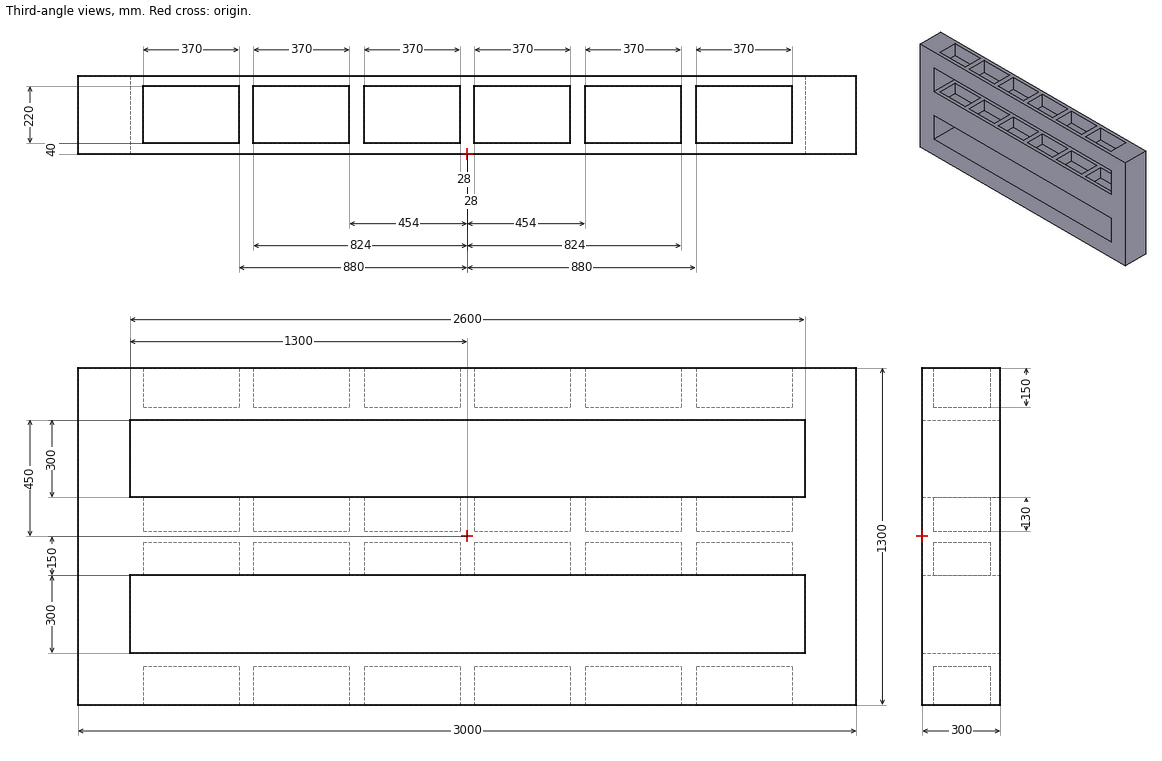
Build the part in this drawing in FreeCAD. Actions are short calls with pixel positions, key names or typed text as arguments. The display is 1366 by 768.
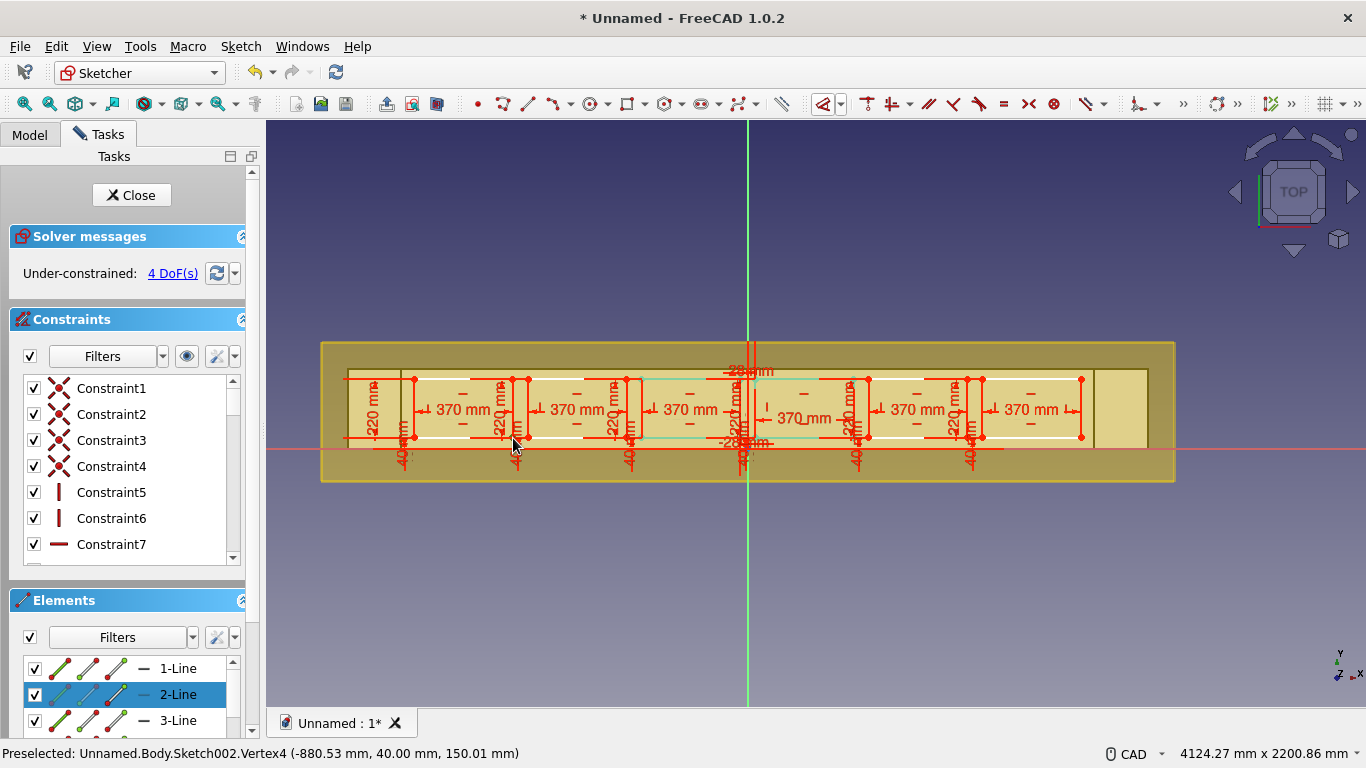
key(l)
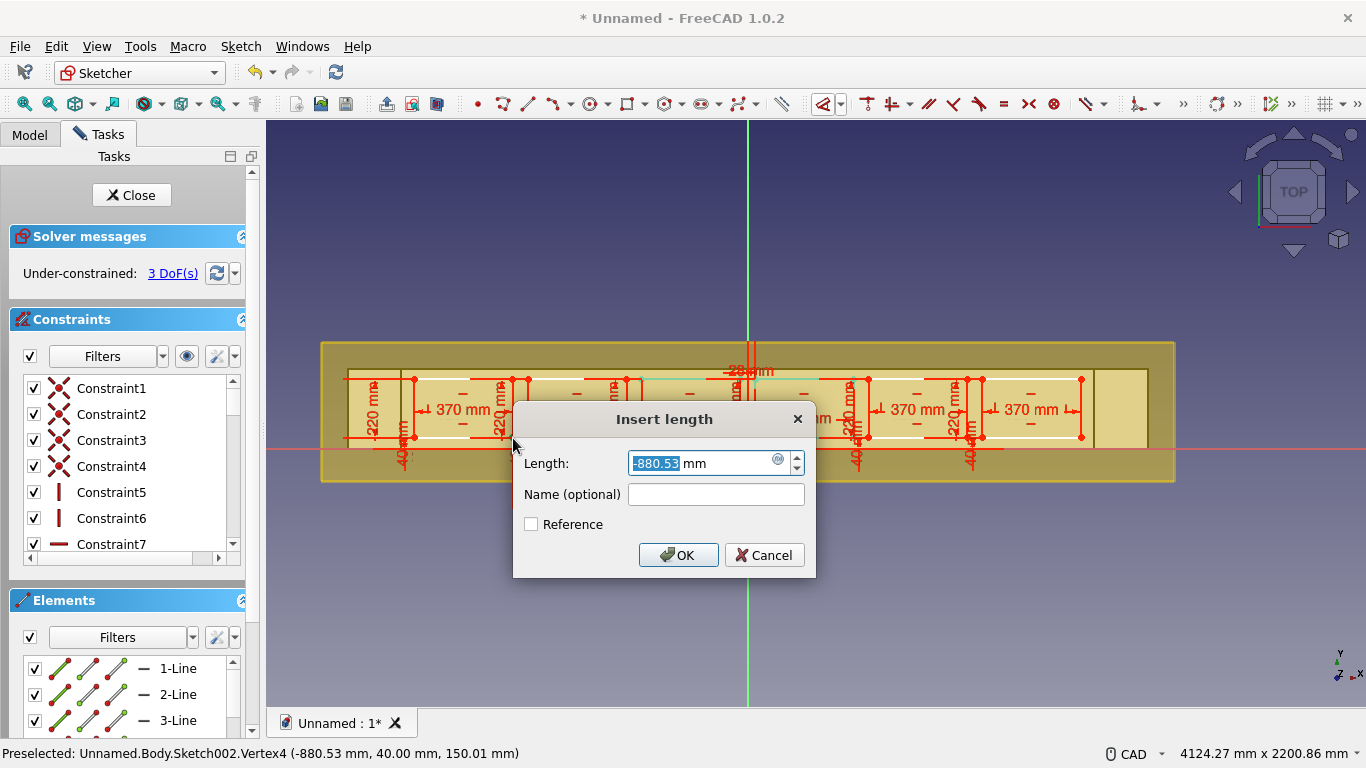
text(-880)
key(Return)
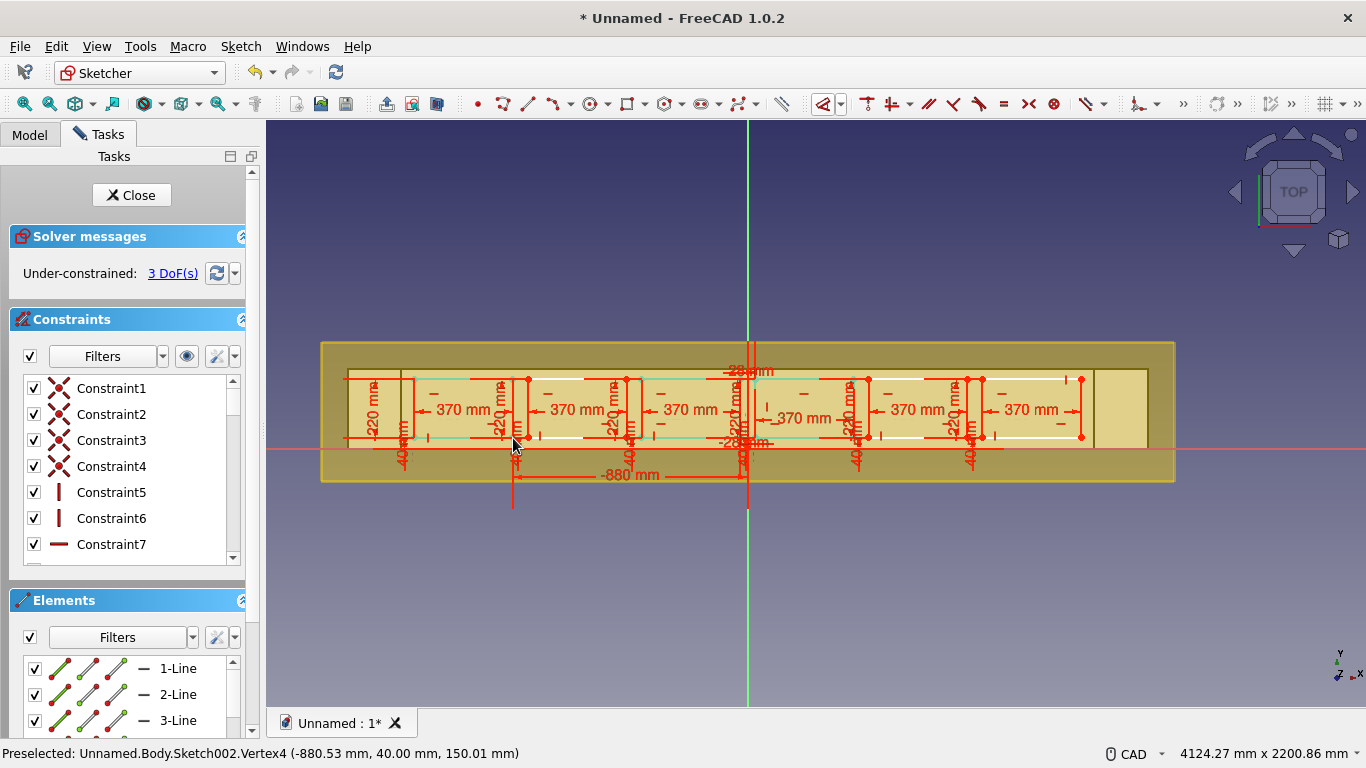
click(528, 379)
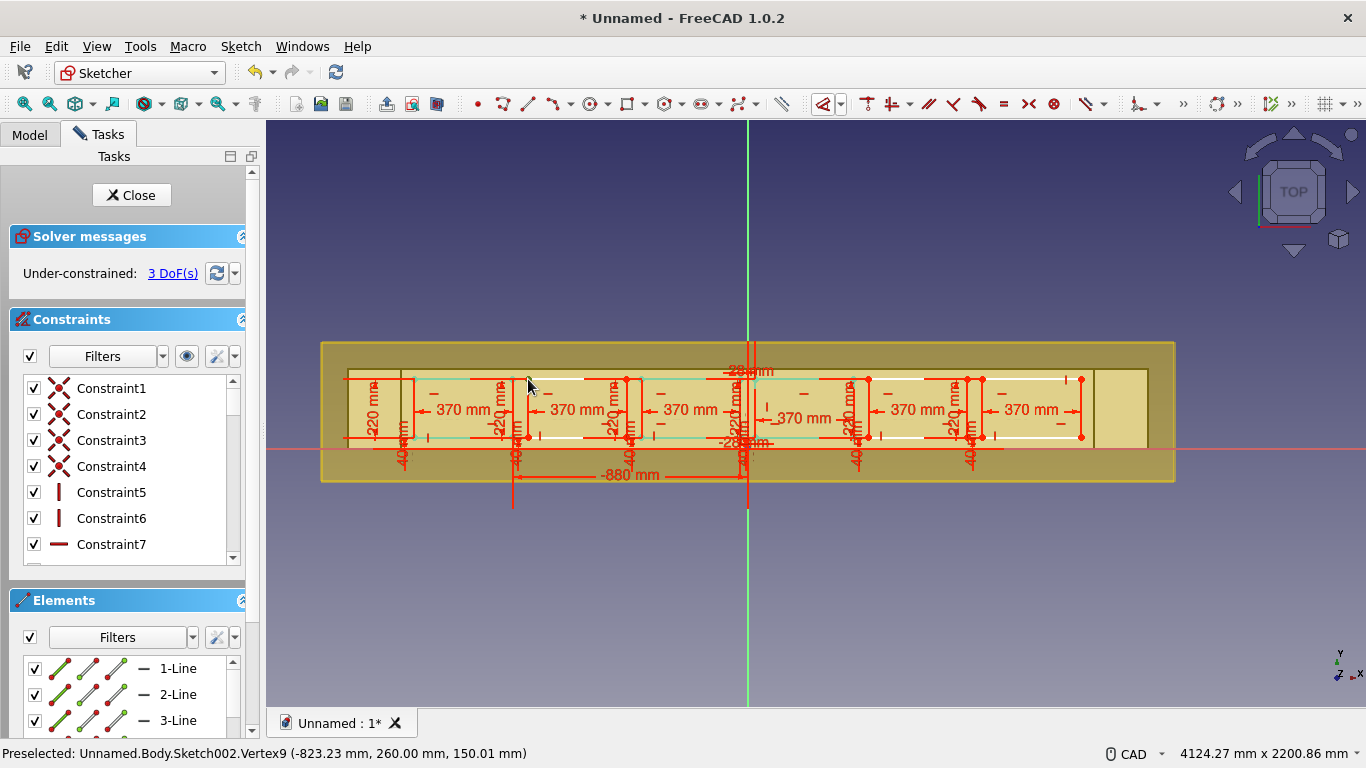
key(l)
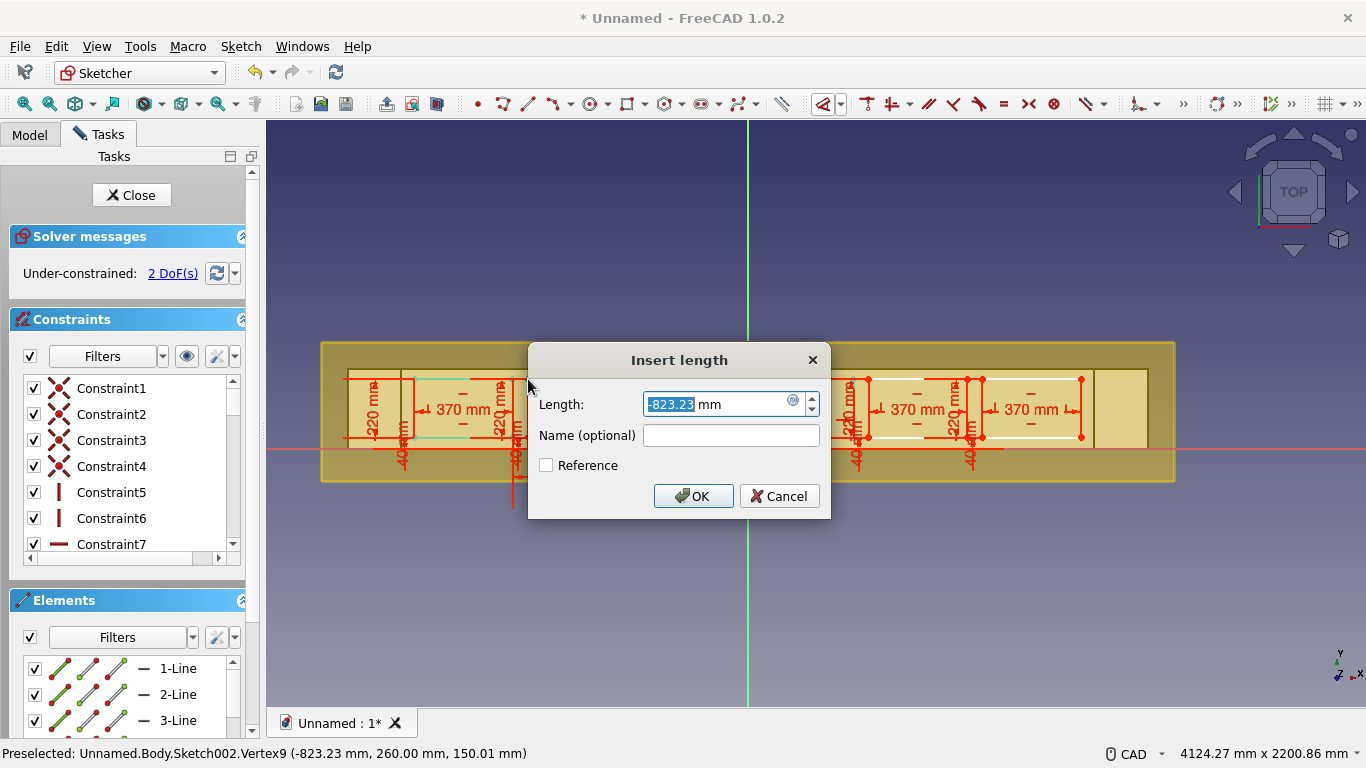
text(-824)
key(Return)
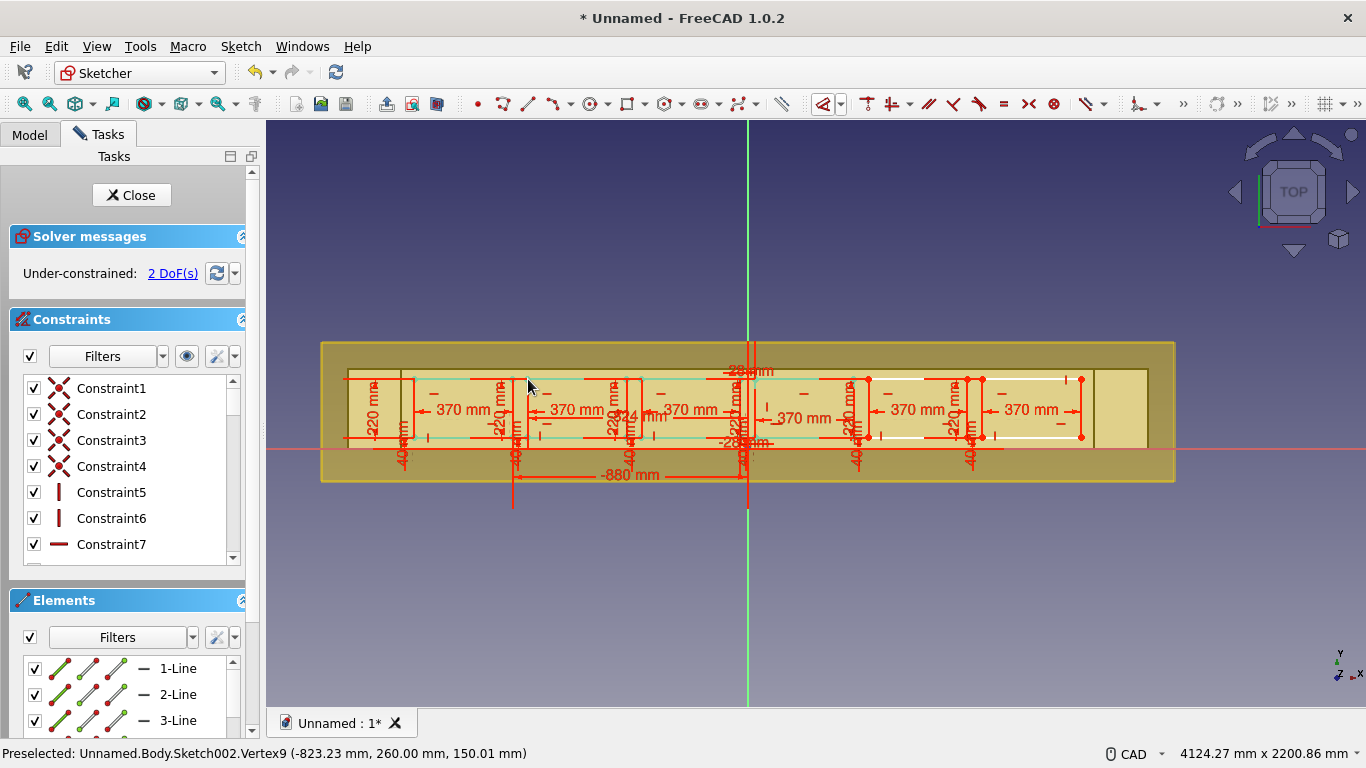
click(869, 379)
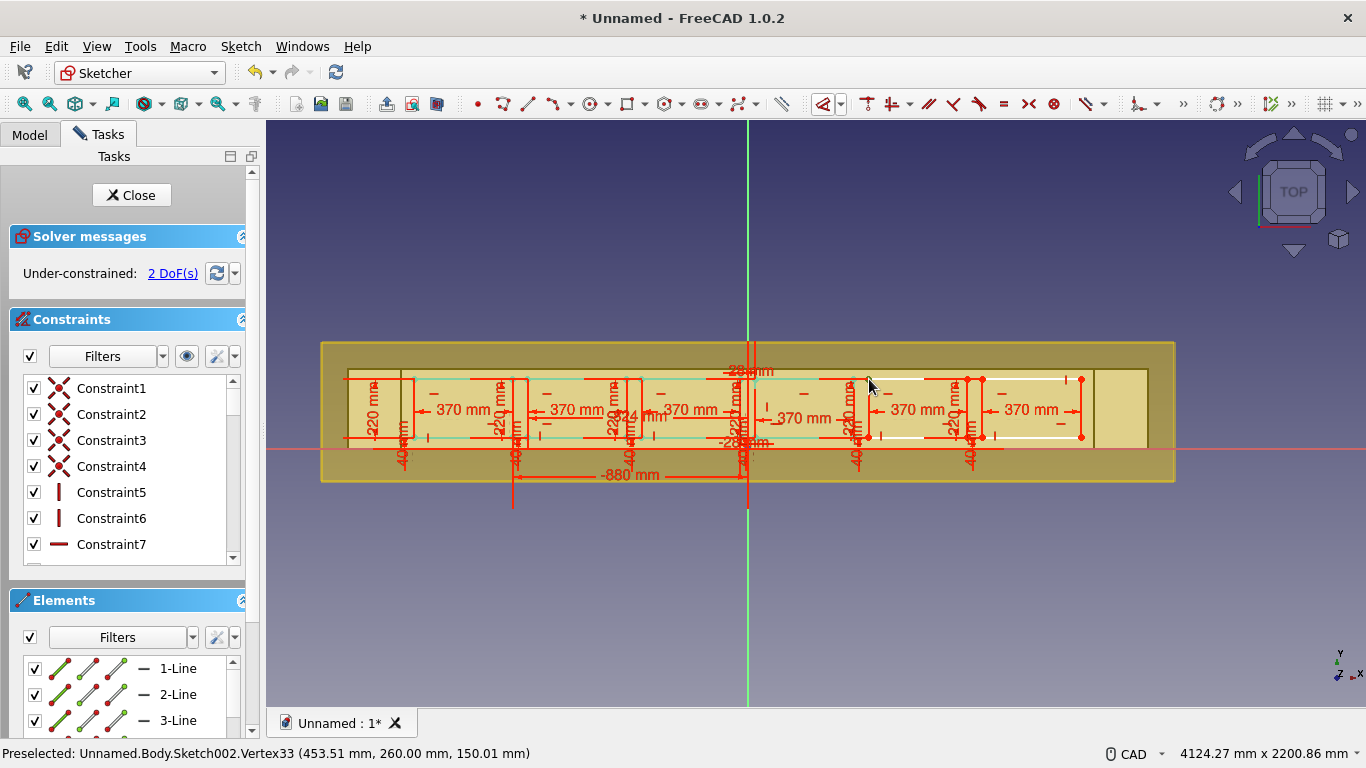
click(840, 104)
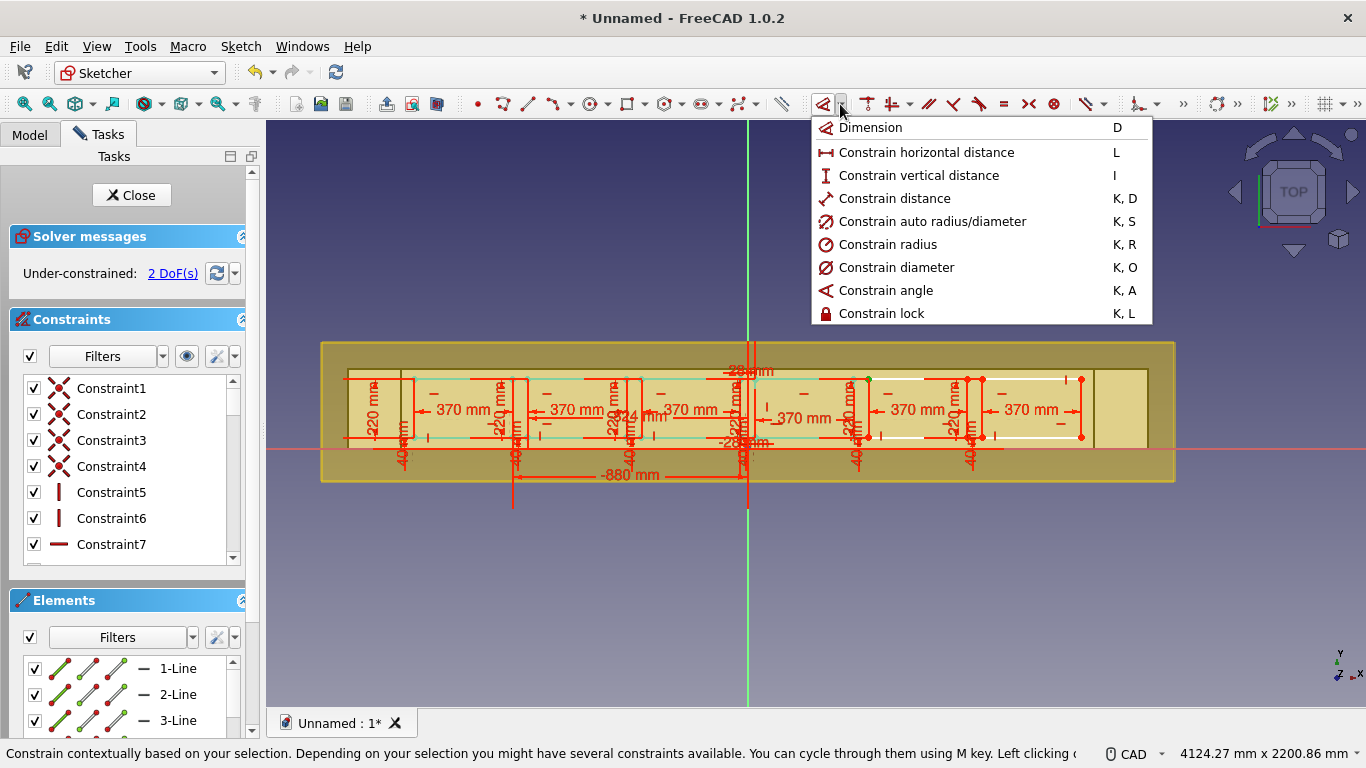
click(982, 152)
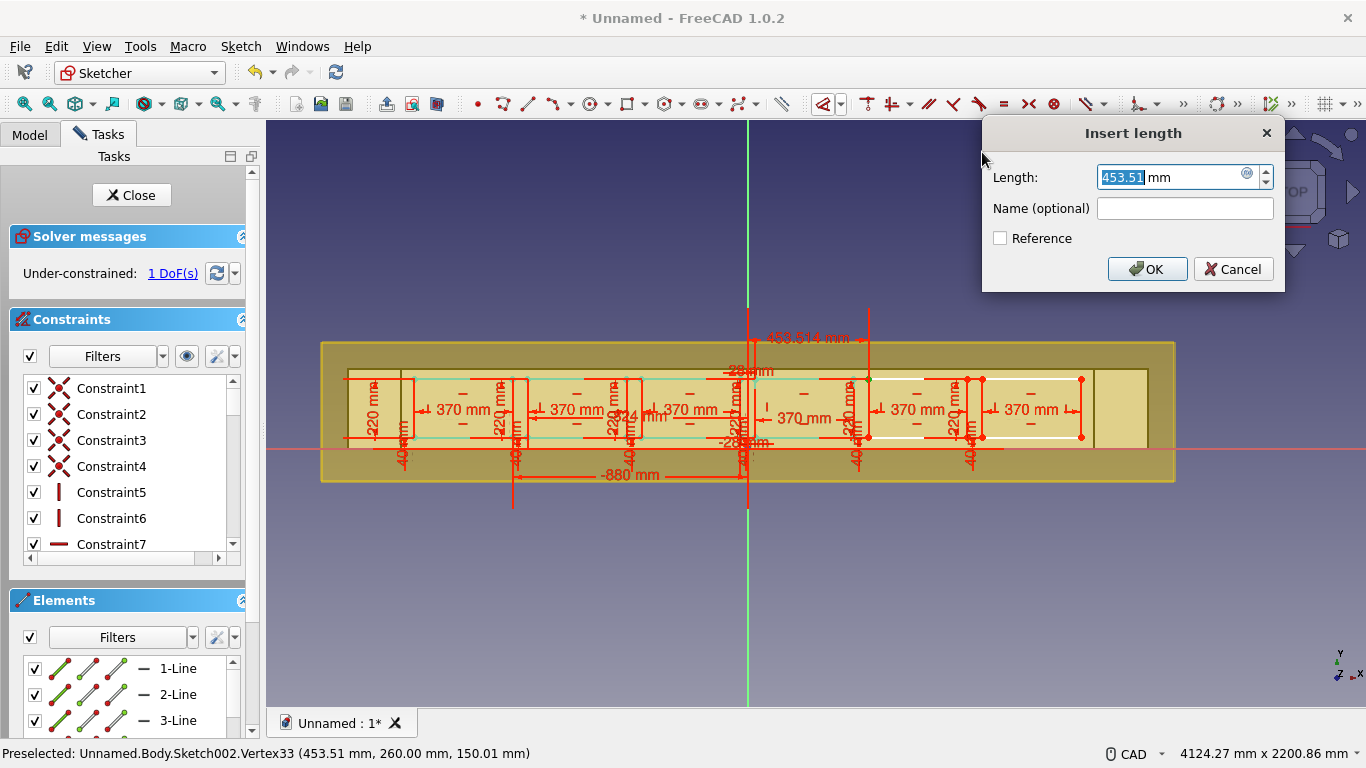
text(454)
key(Return)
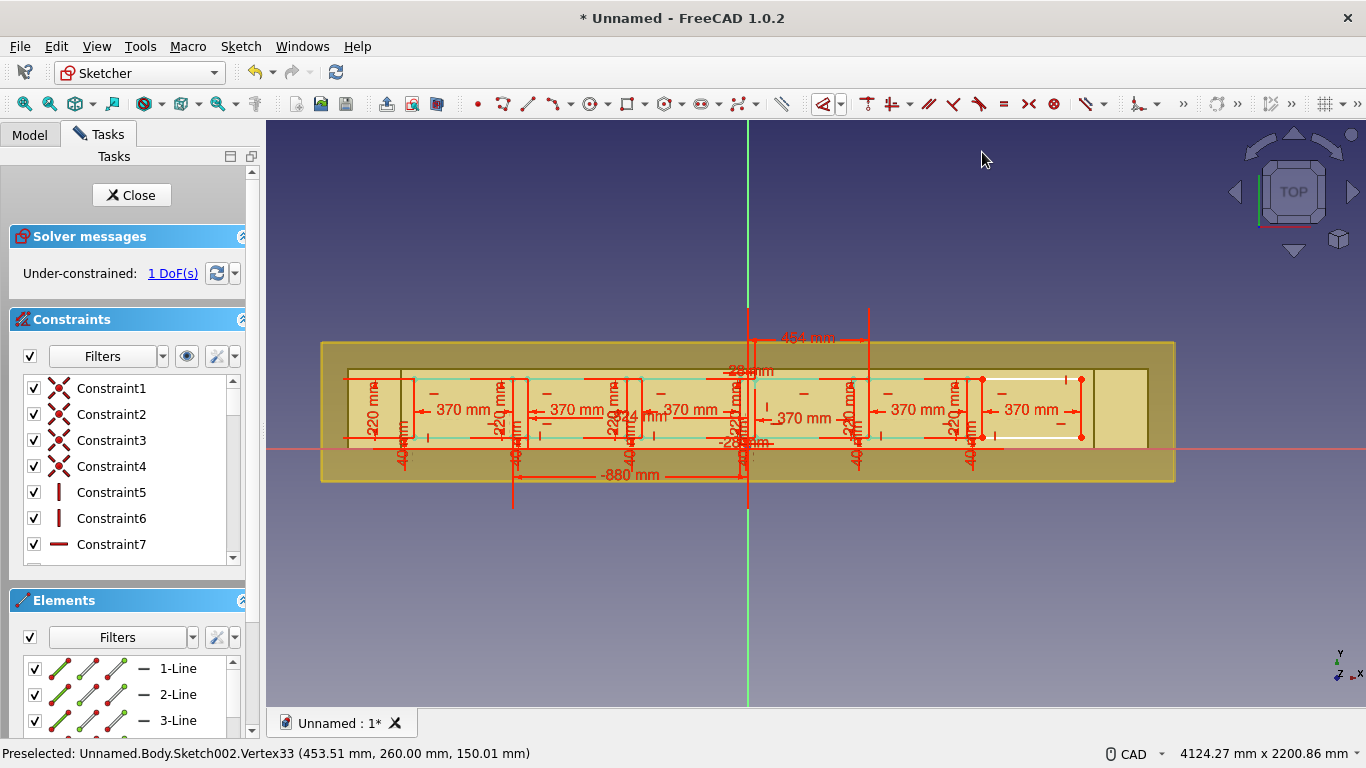
click(982, 379)